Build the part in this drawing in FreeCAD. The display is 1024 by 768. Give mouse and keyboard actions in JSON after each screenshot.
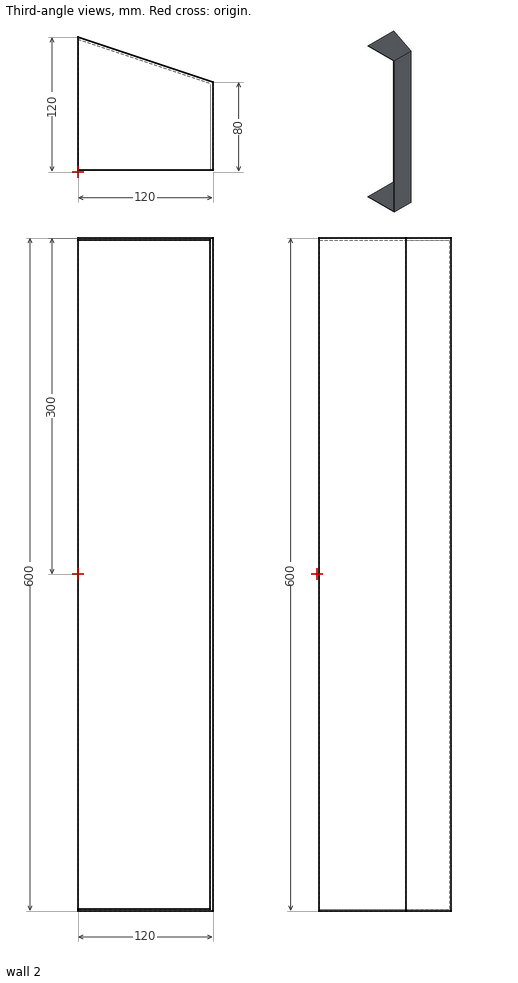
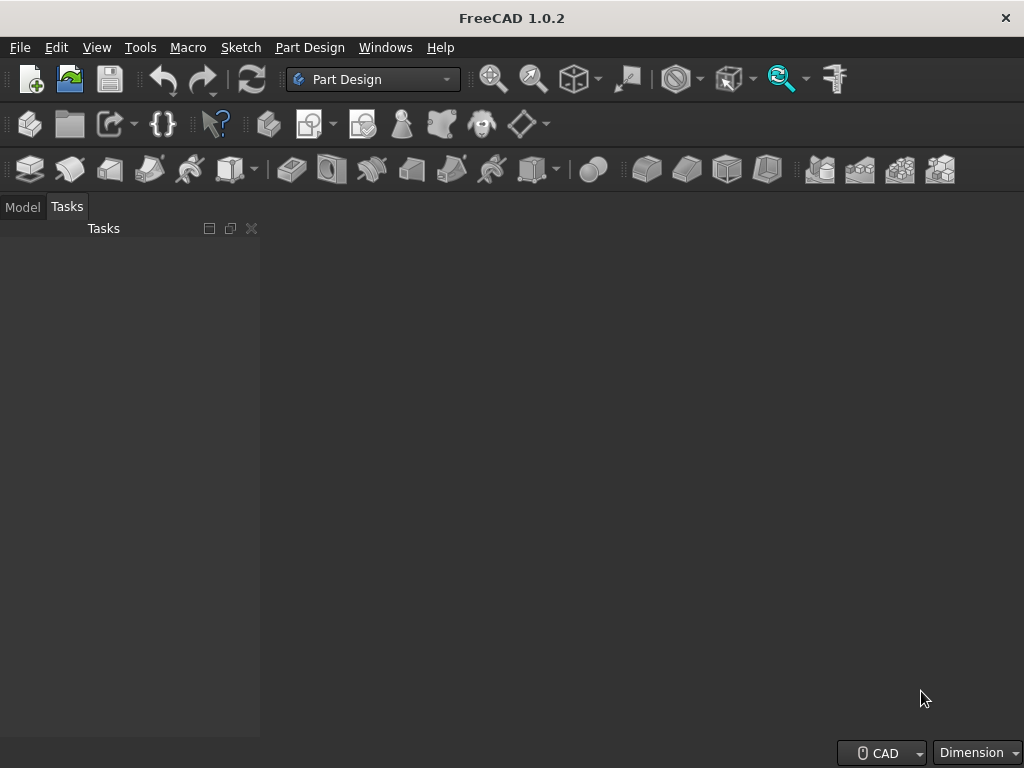
{"action": "left_click", "coordinate": [30, 80]}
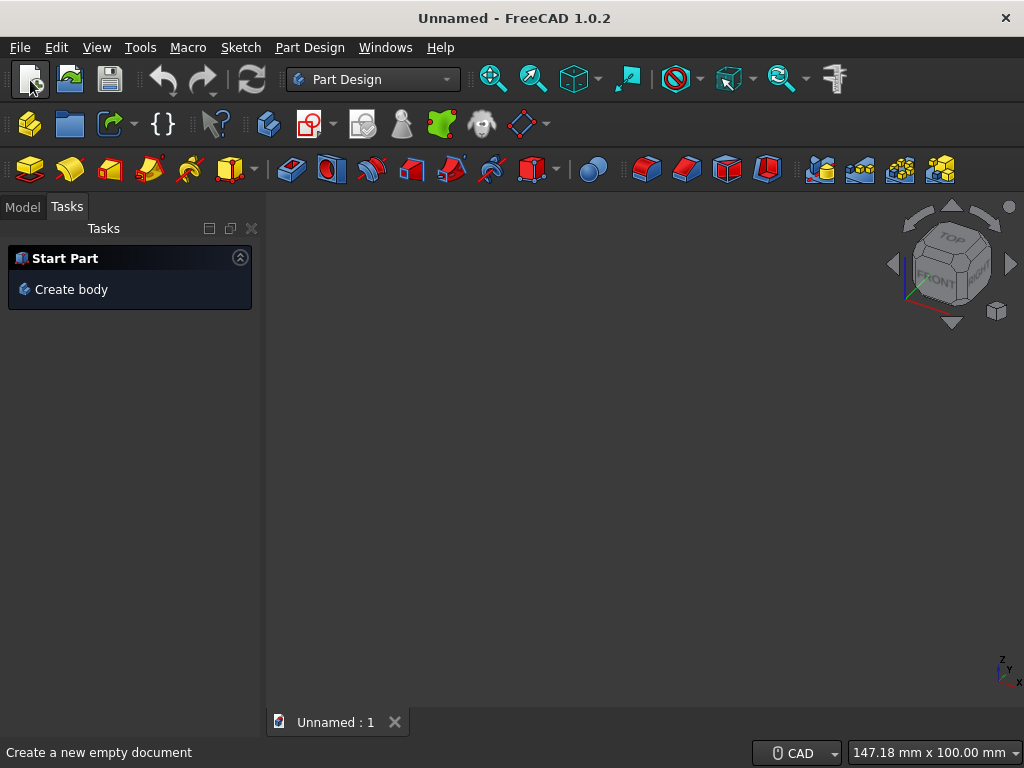
{"action": "left_click", "coordinate": [310, 124]}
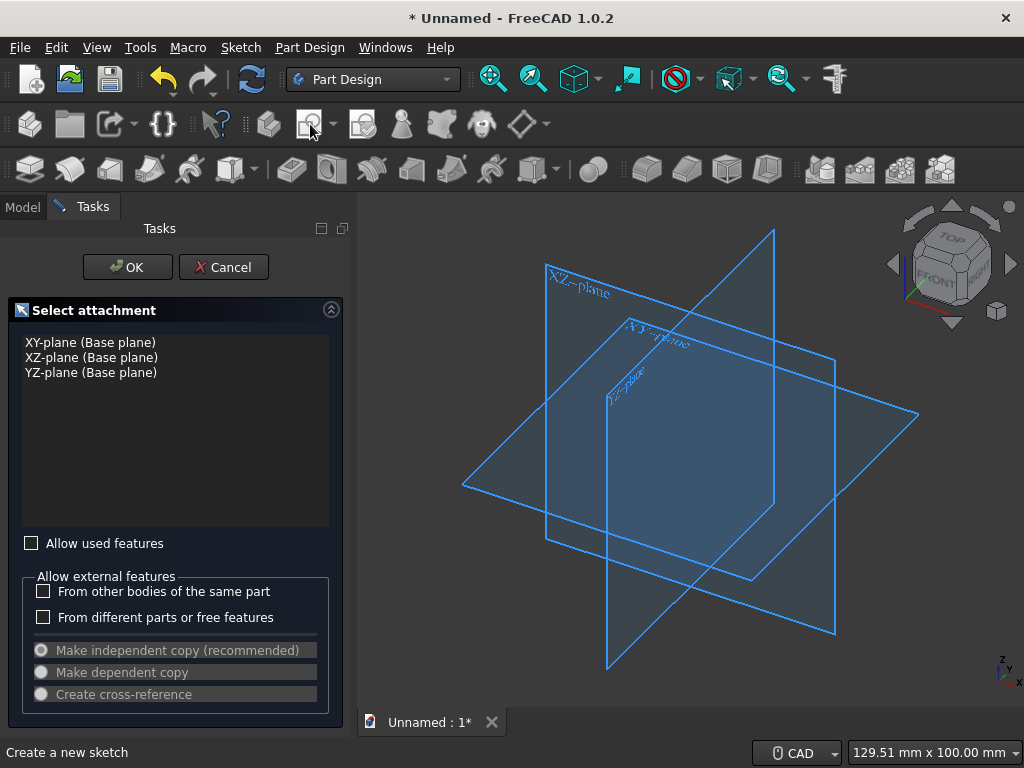
{"action": "left_click", "coordinate": [82, 342]}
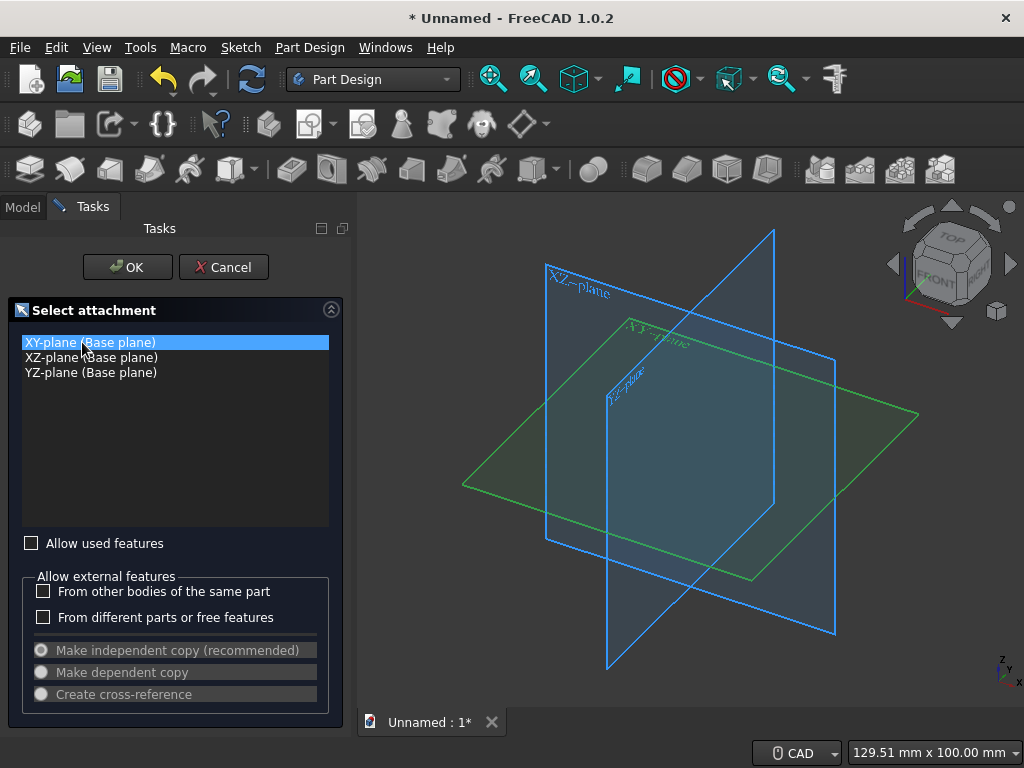
{"action": "left_click", "coordinate": [128, 267]}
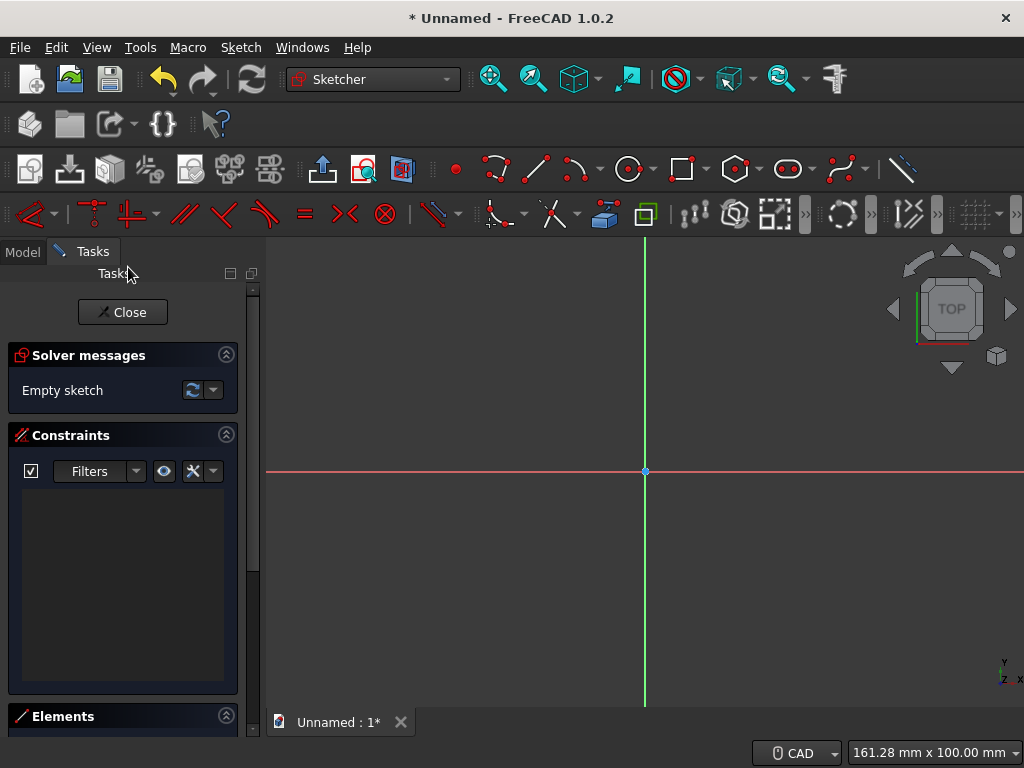
{"action": "scroll", "coordinate": [294, 679], "scroll_direction": "down", "scroll_amount": 4}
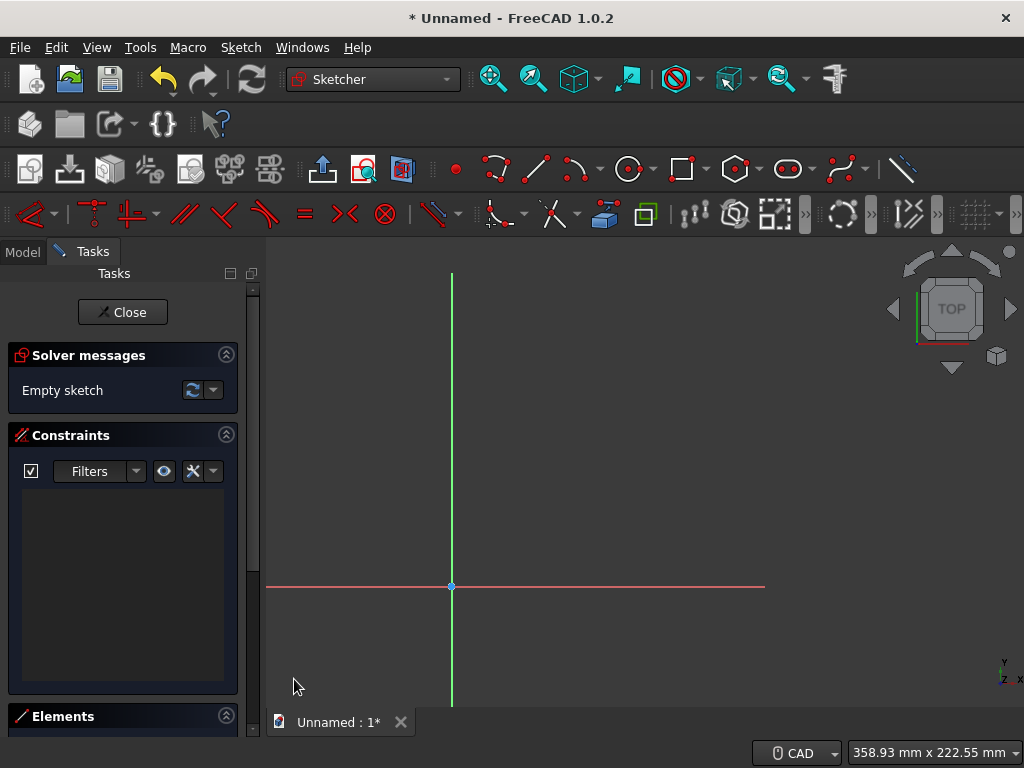
{"action": "left_click", "coordinate": [496, 170]}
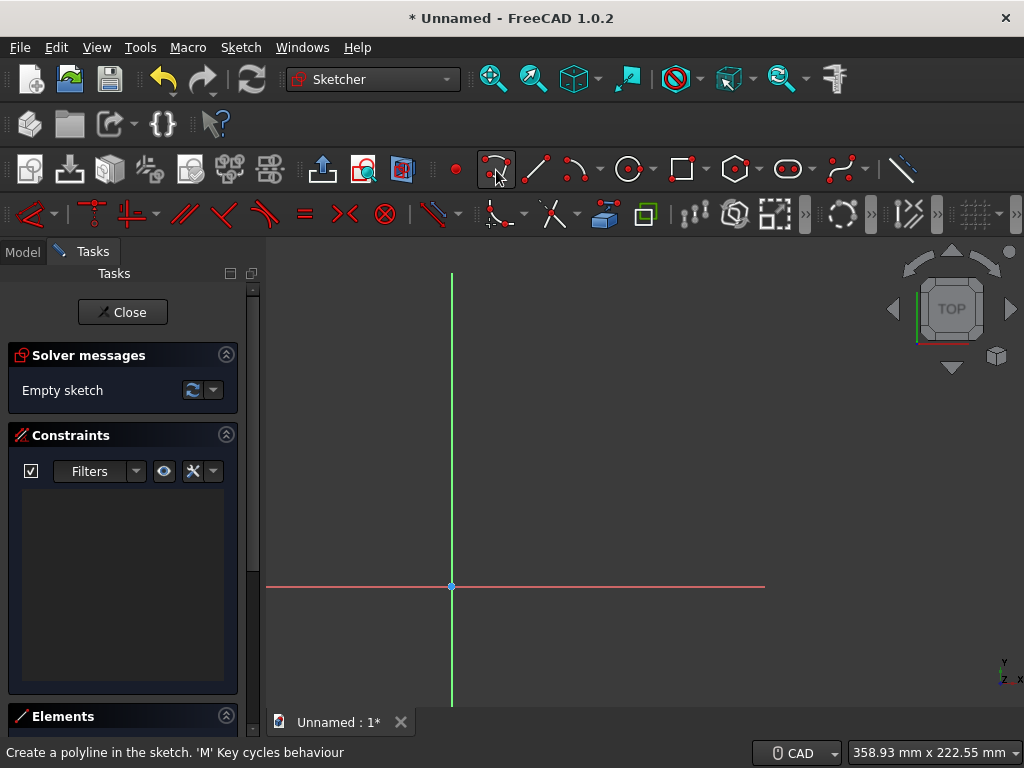
{"action": "left_click", "coordinate": [452, 587]}
{"action": "left_click", "coordinate": [705, 578]}
{"action": "left_click", "coordinate": [705, 418]}
{"action": "left_click", "coordinate": [461, 333]}
{"action": "left_click", "coordinate": [452, 587]}
{"action": "key", "text": "Escape"}
{"action": "key", "text": "Escape"}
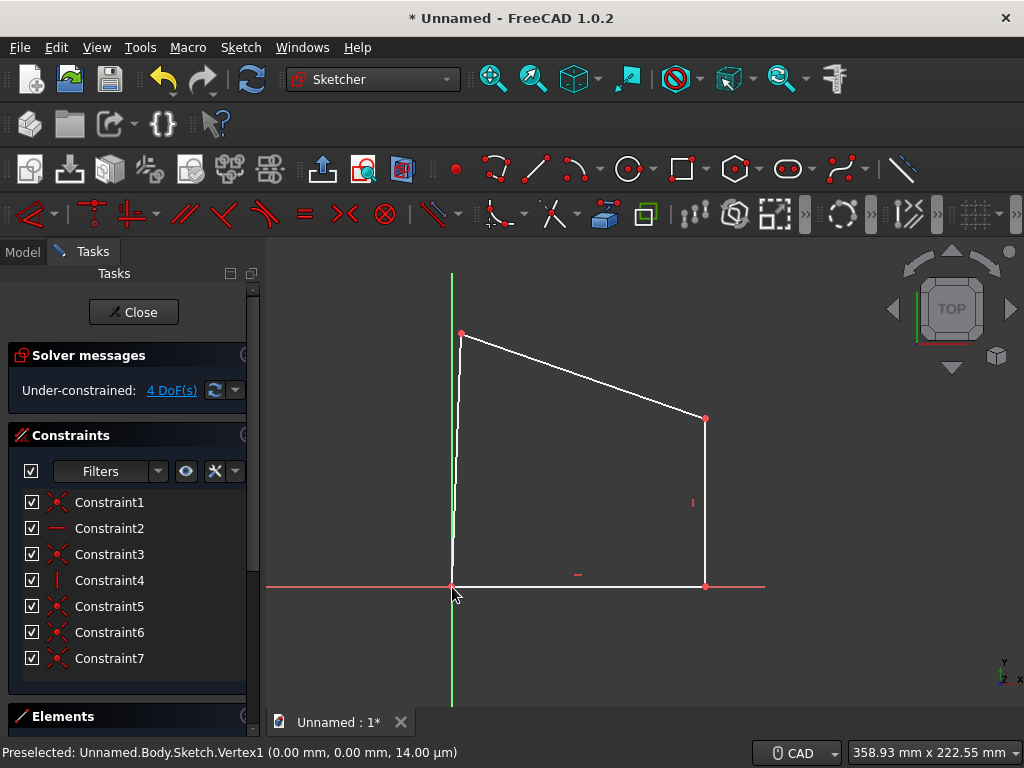
{"action": "left_click", "coordinate": [455, 511]}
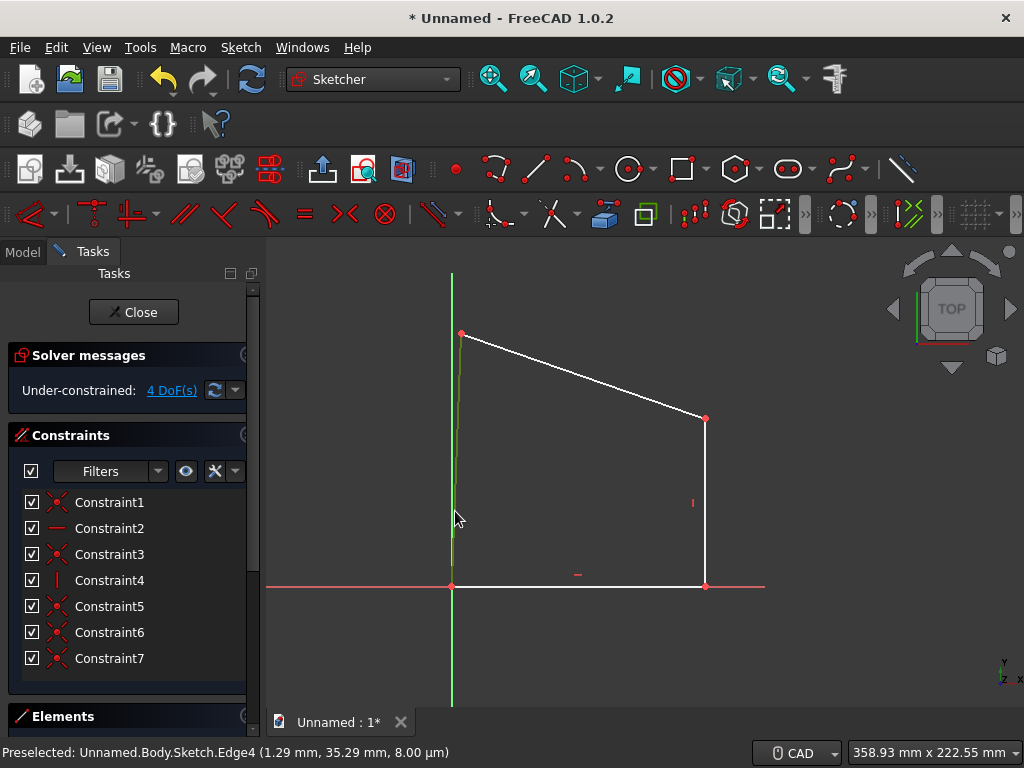
{"action": "left_click", "coordinate": [158, 214]}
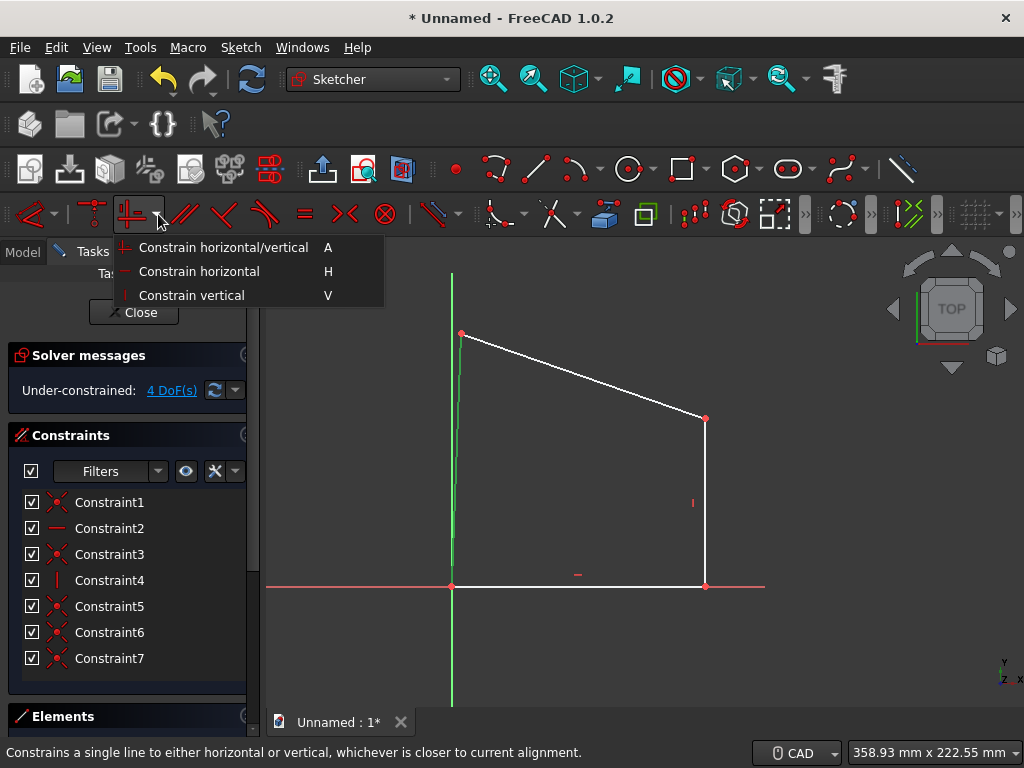
{"action": "left_click", "coordinate": [249, 295]}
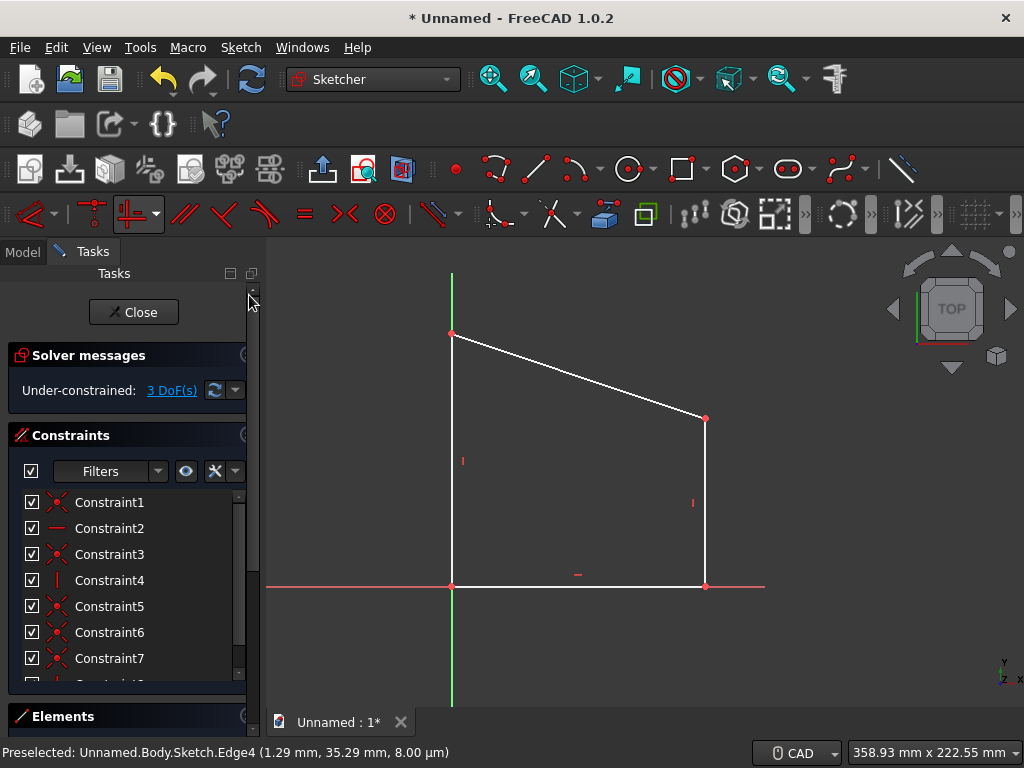
{"action": "left_click", "coordinate": [705, 536]}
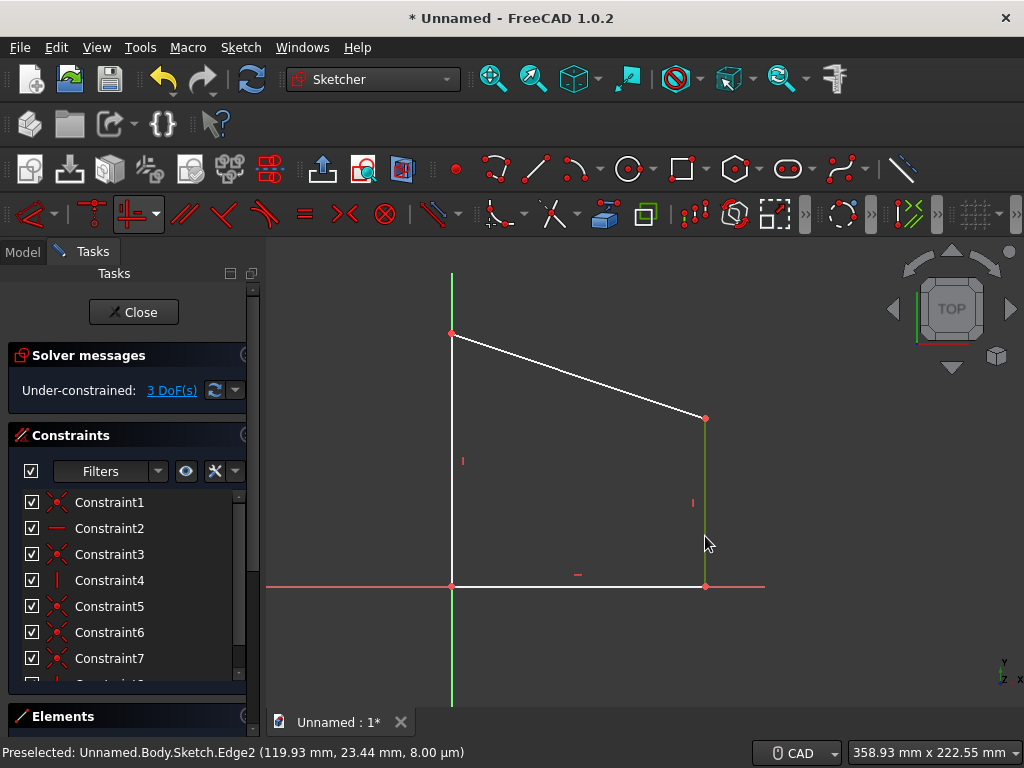
{"action": "left_click", "coordinate": [56, 214]}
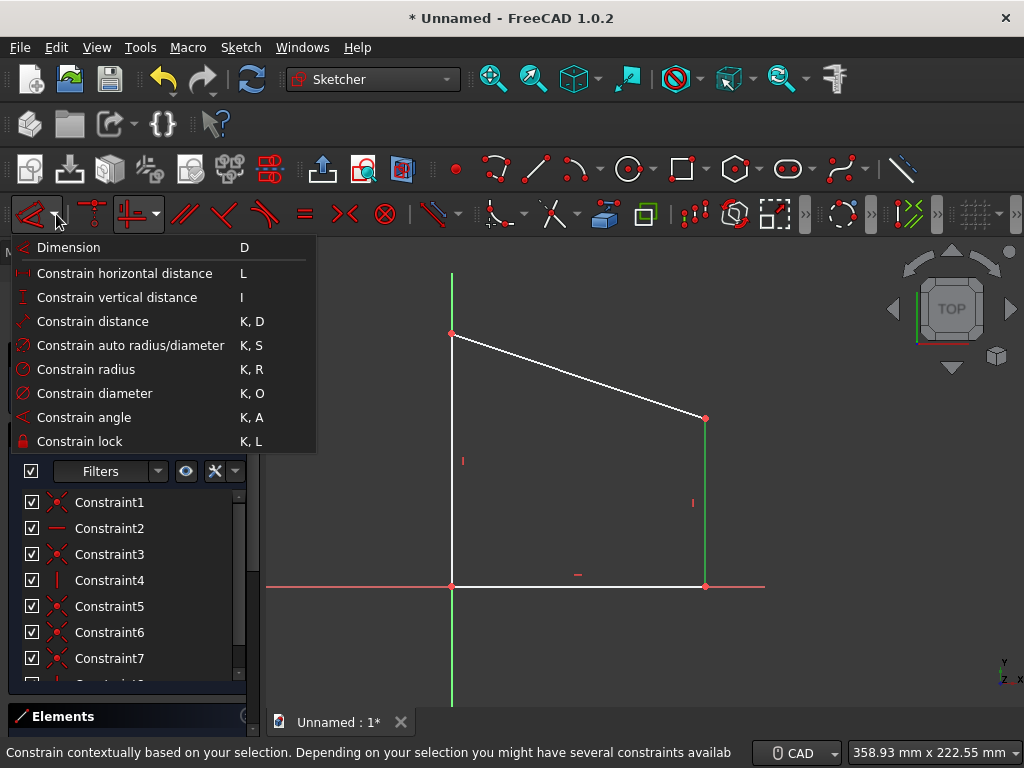
{"action": "left_click", "coordinate": [164, 297]}